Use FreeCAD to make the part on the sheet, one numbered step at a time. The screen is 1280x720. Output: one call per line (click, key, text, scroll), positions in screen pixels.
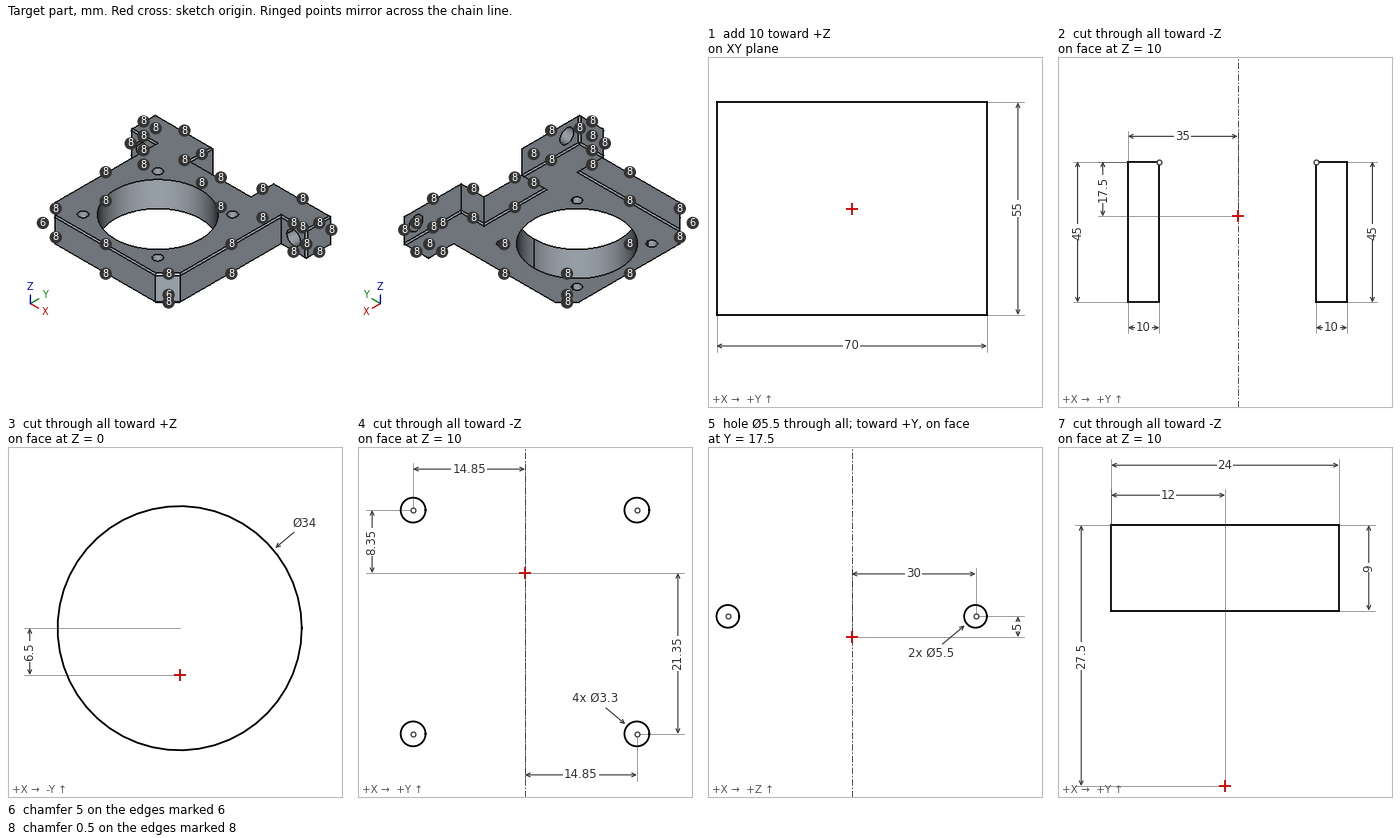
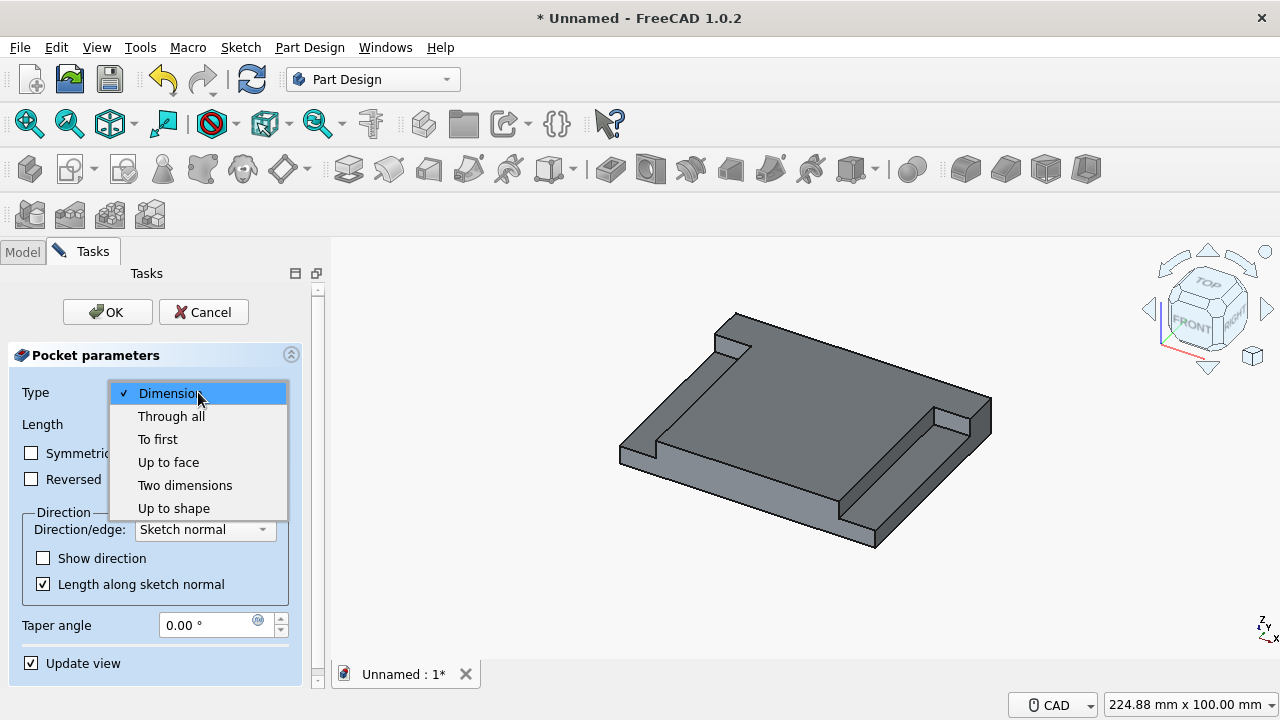
click(198, 416)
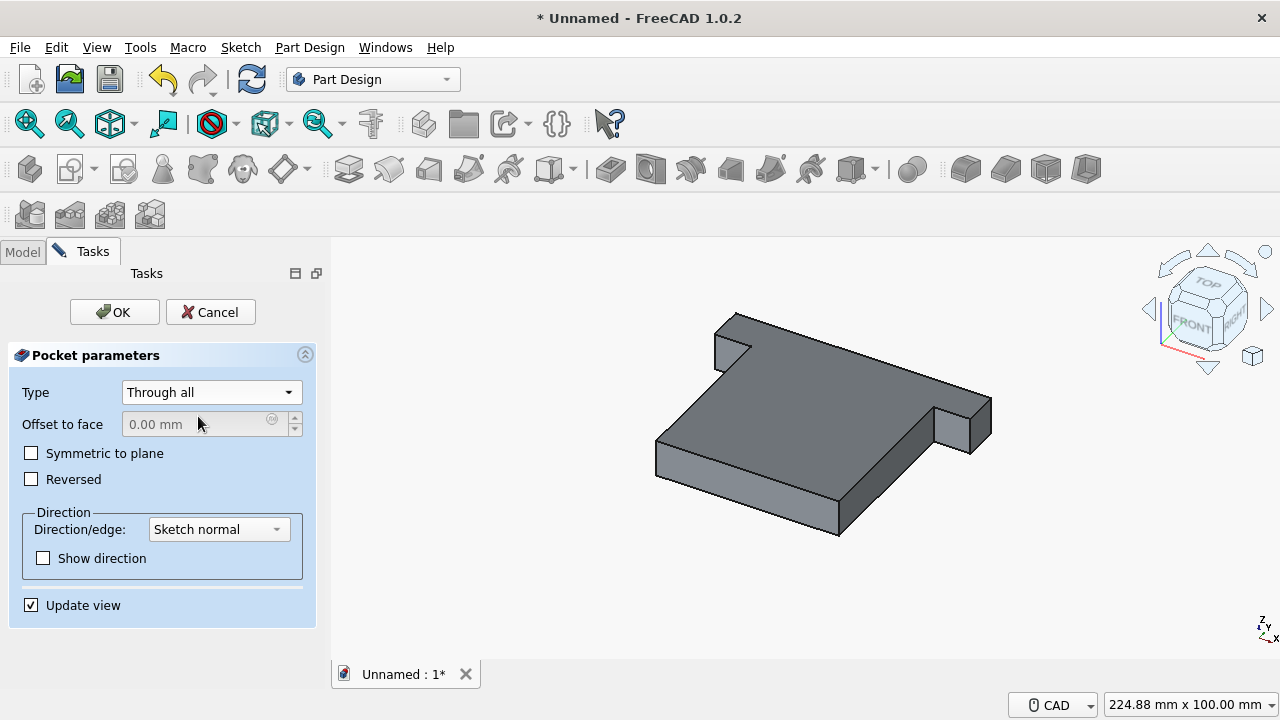
click(115, 312)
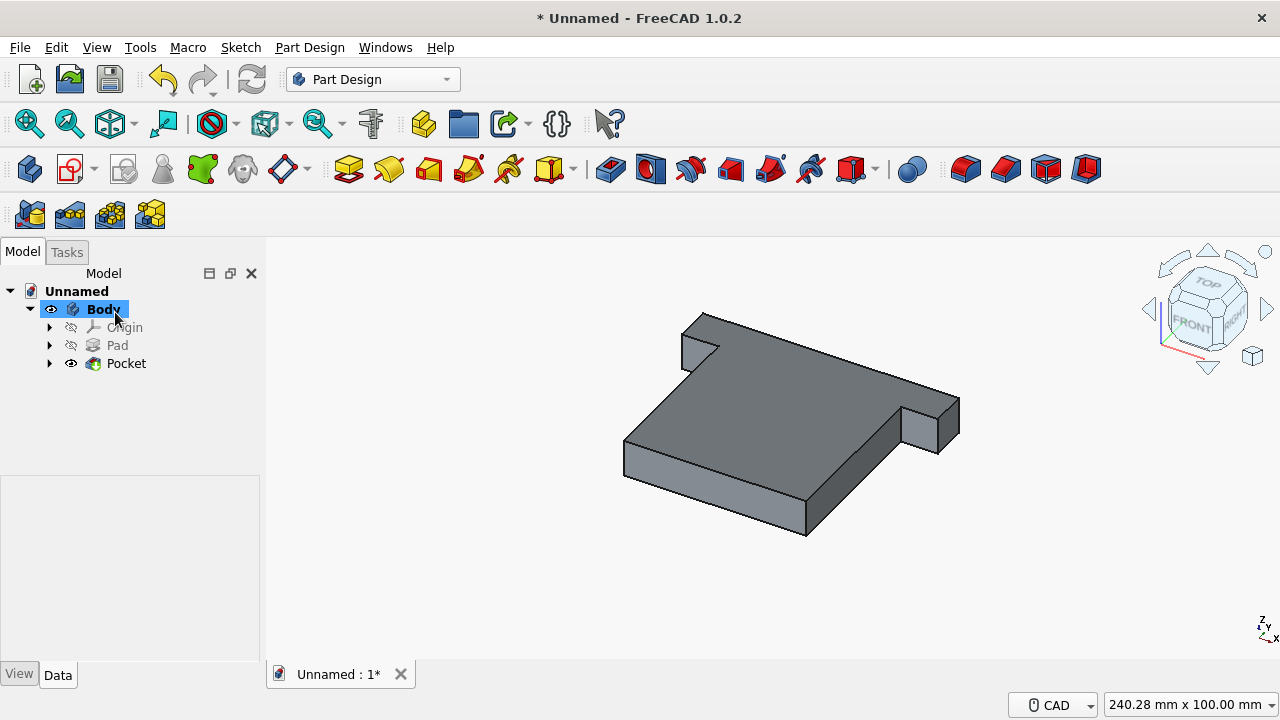
key(5)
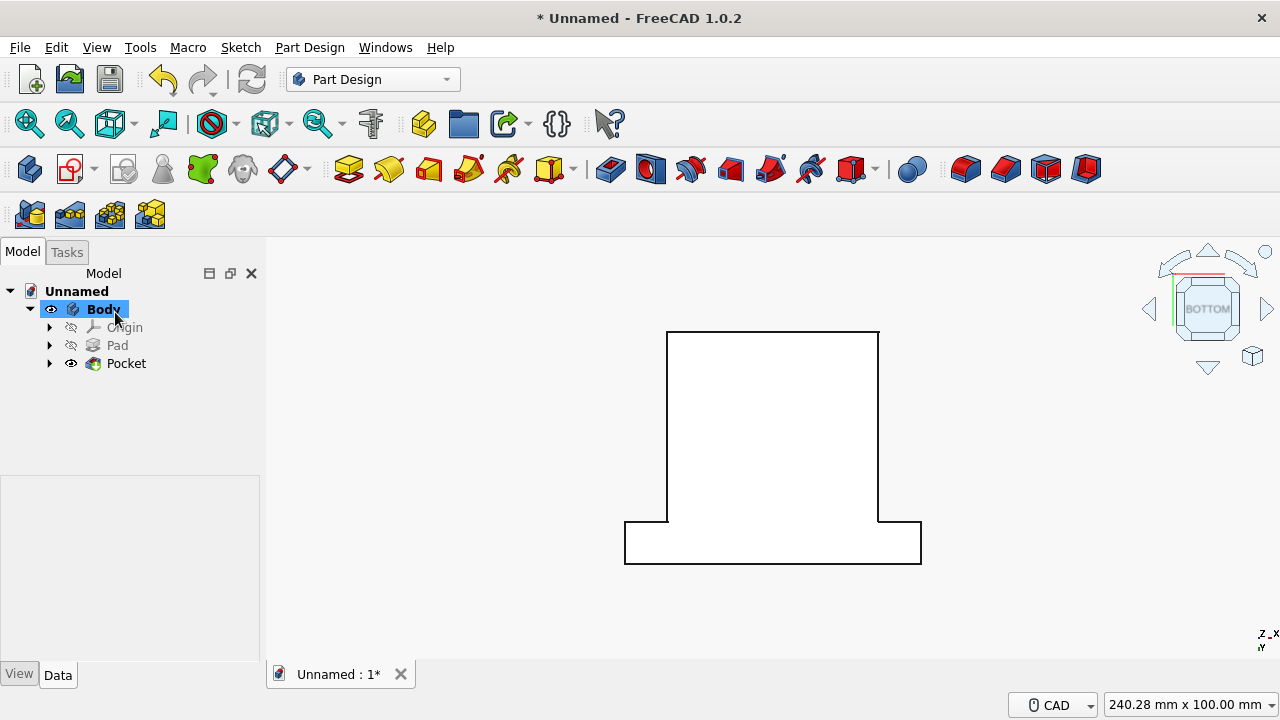
click(773, 447)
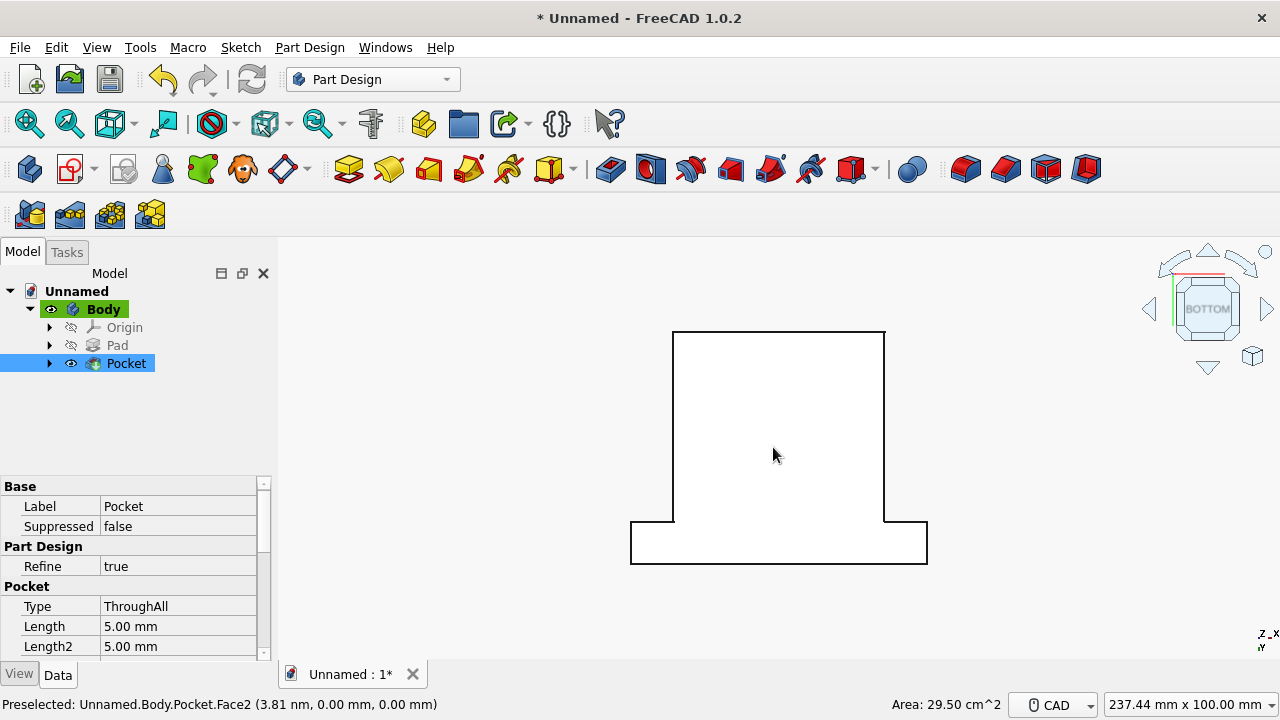
click(70, 170)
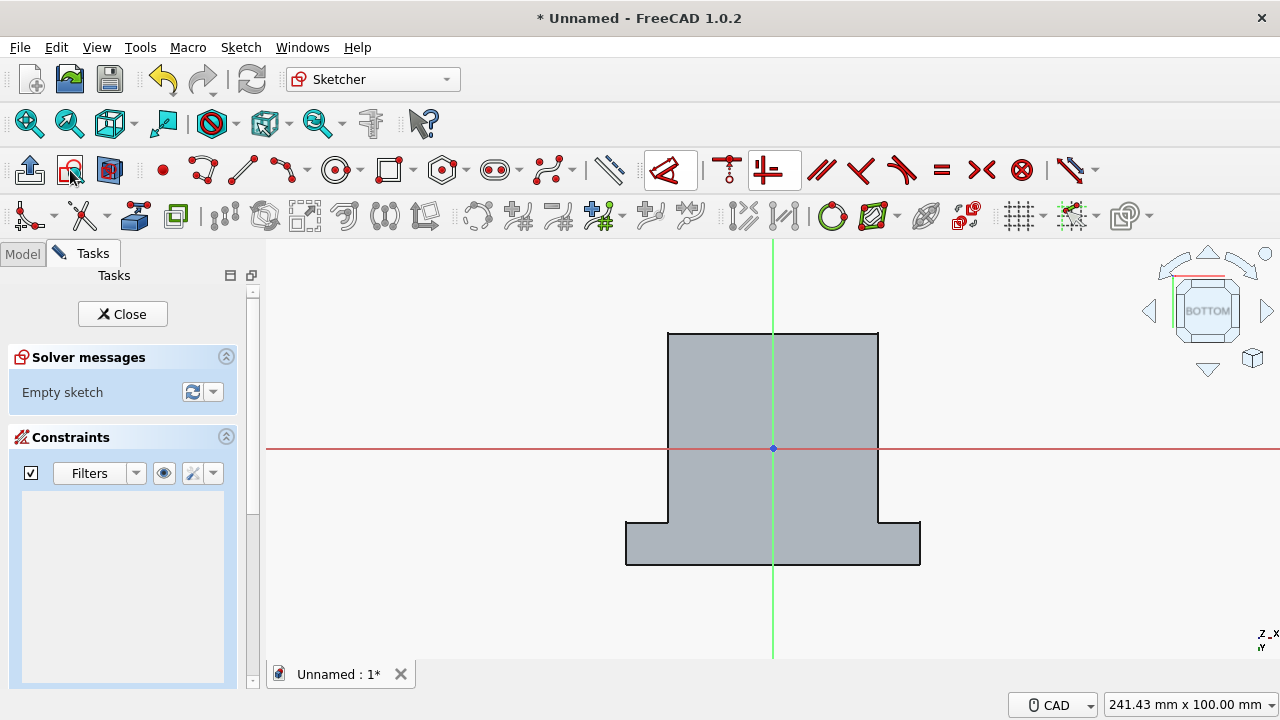
scroll(856, 388, up, 3)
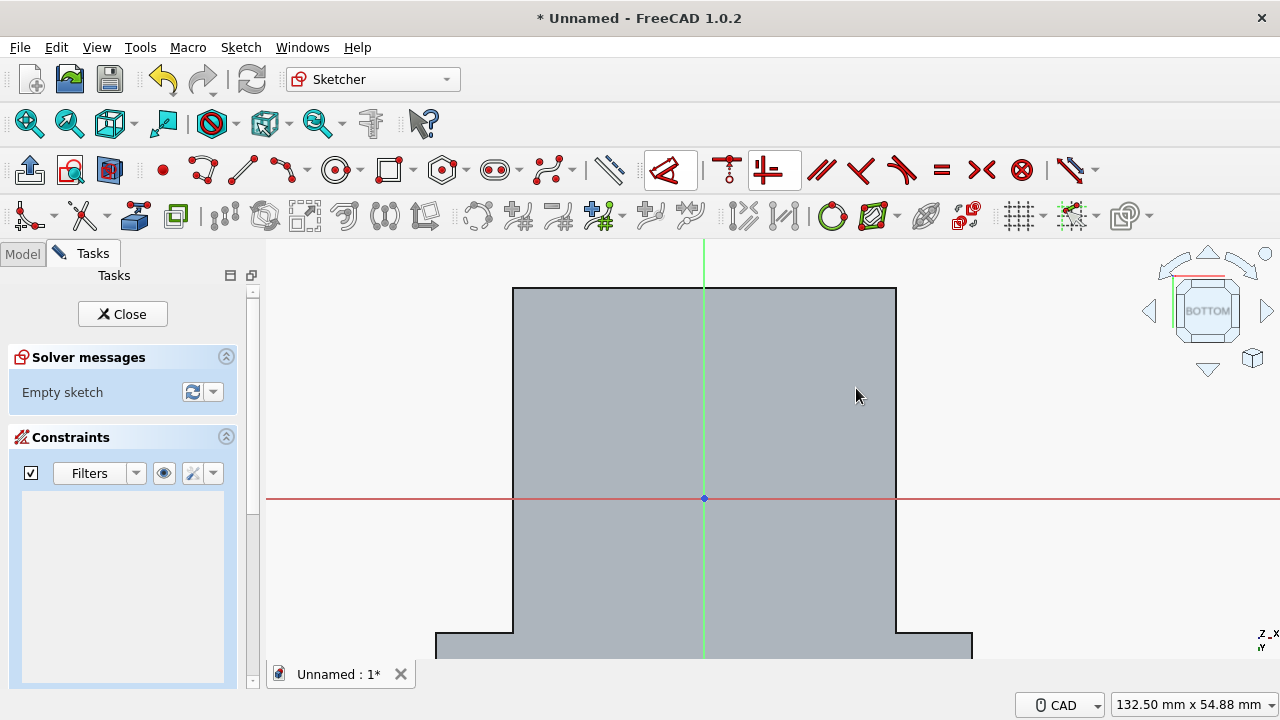
click(336, 170)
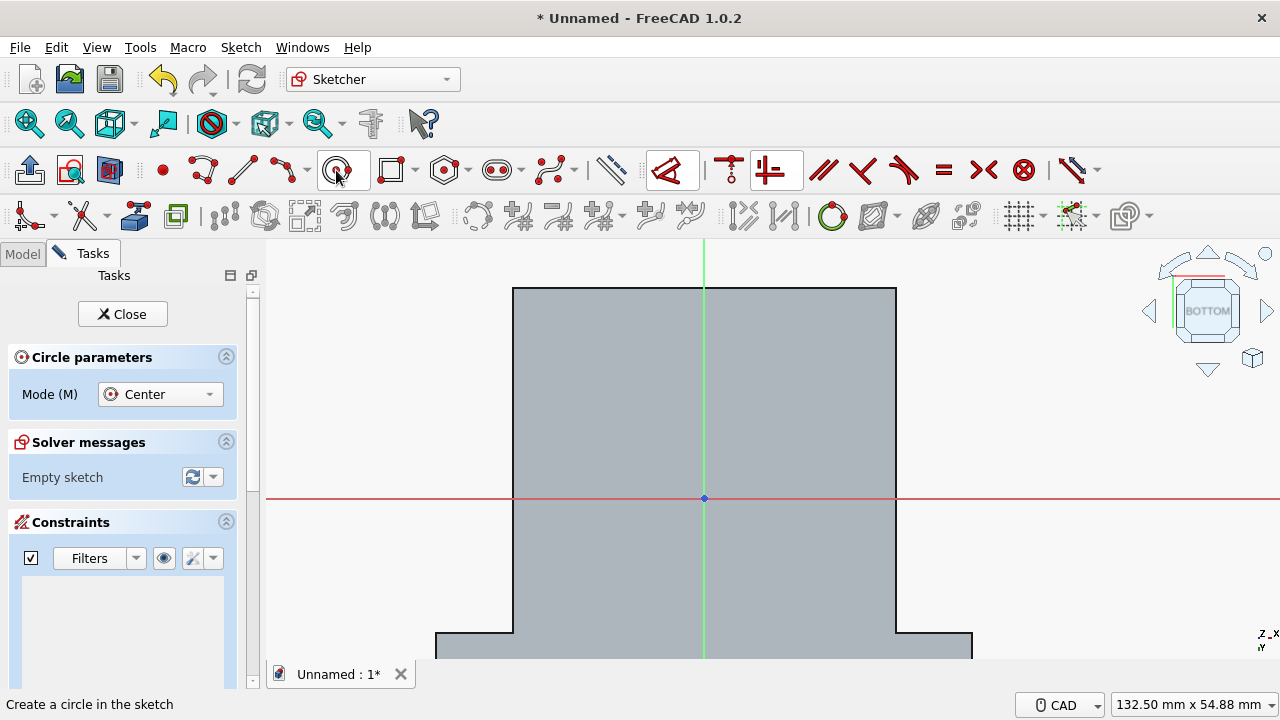
click(704, 449)
move(796, 357)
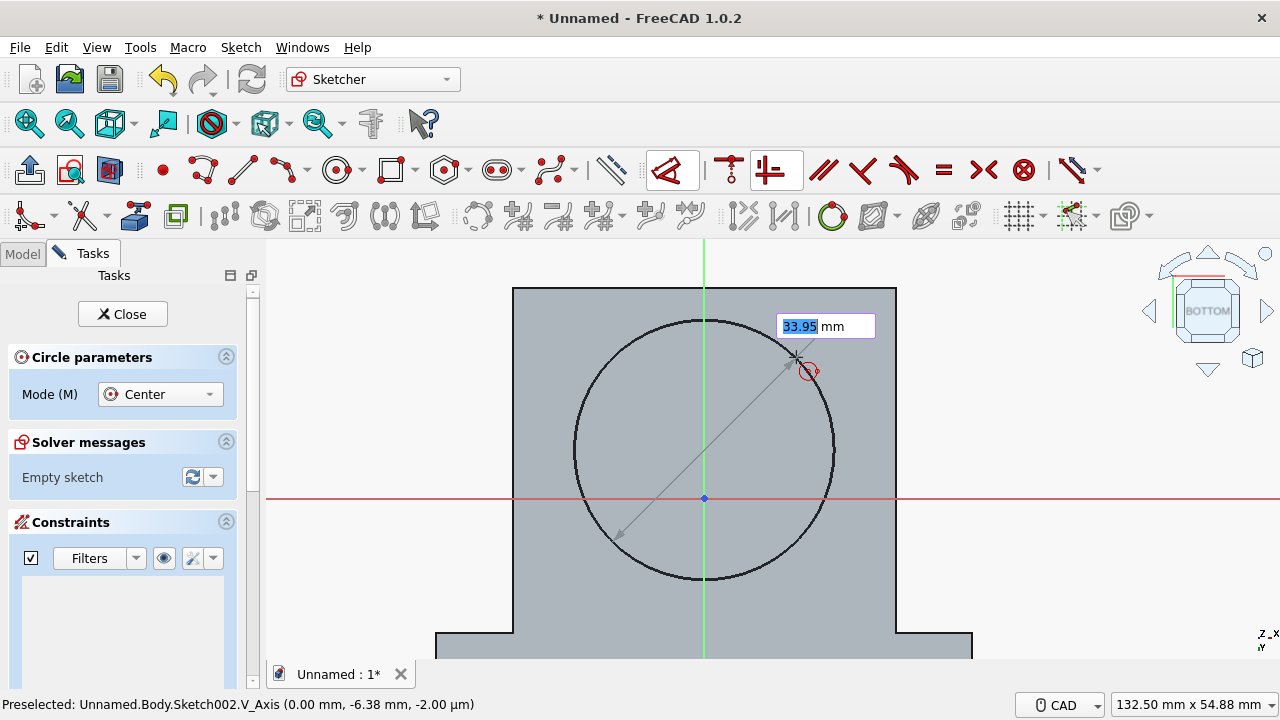
text(34)
key(Return)
key(Escape)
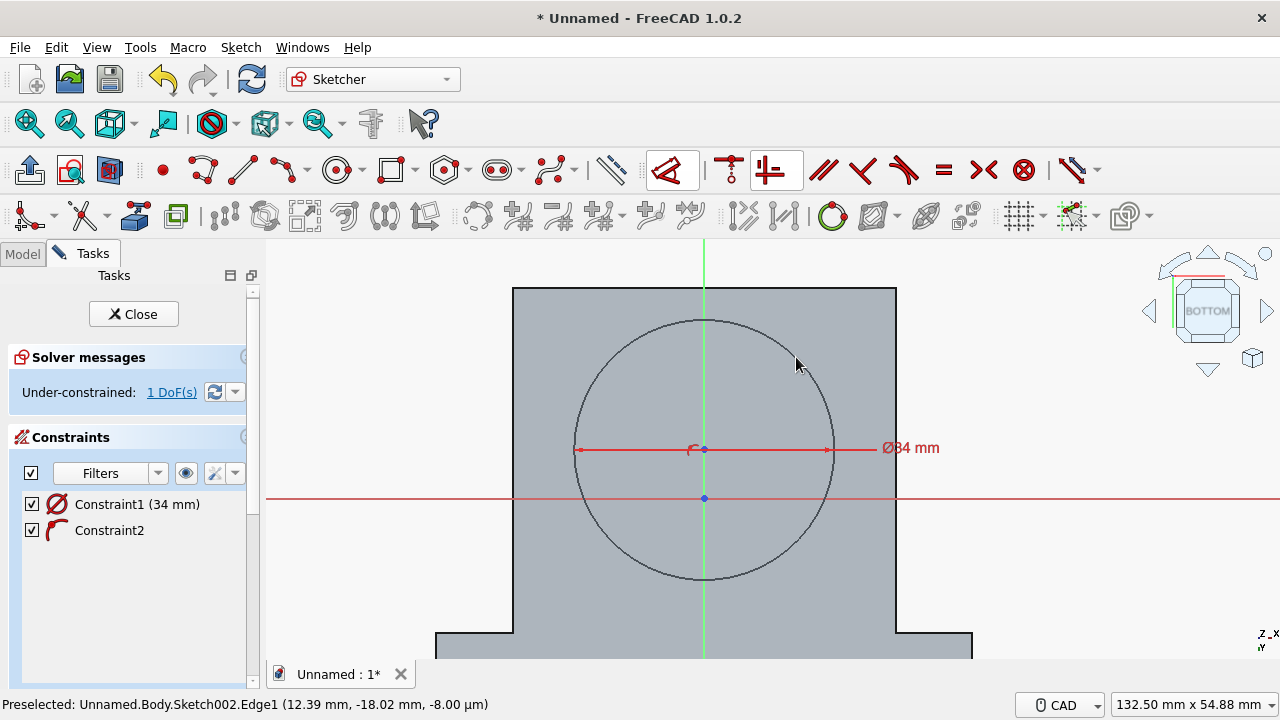
click(704, 450)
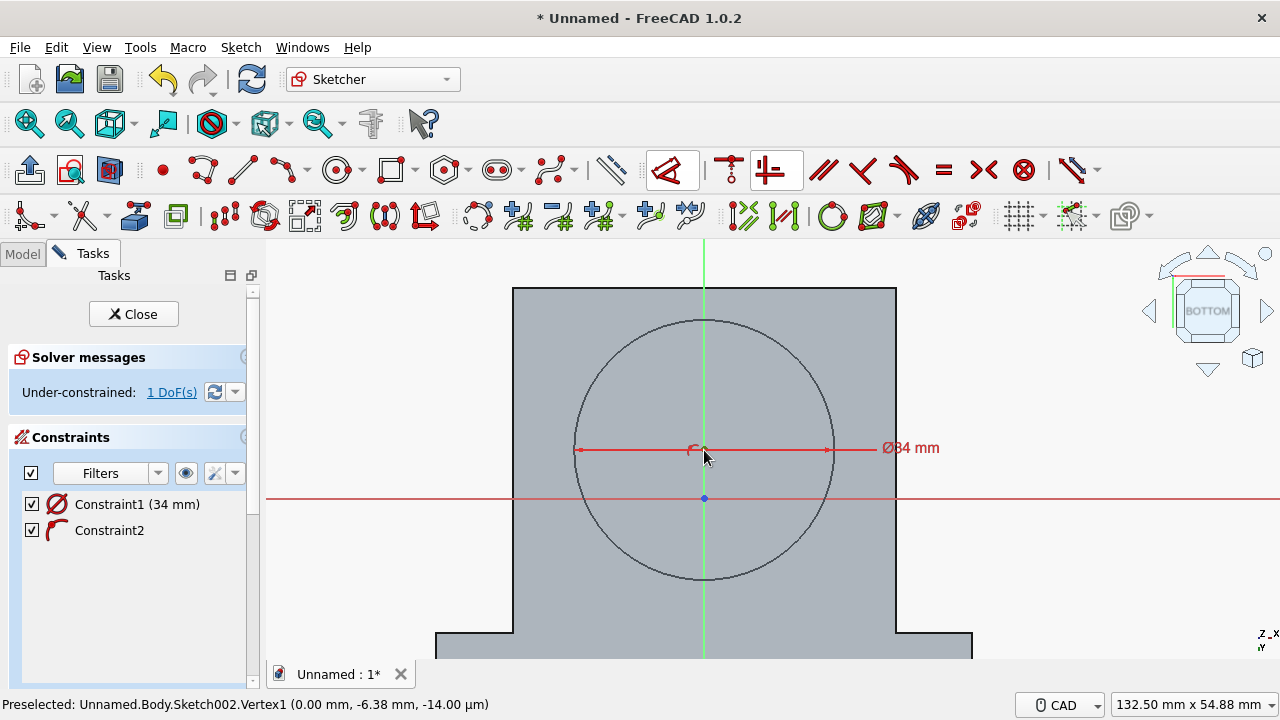
key(i)